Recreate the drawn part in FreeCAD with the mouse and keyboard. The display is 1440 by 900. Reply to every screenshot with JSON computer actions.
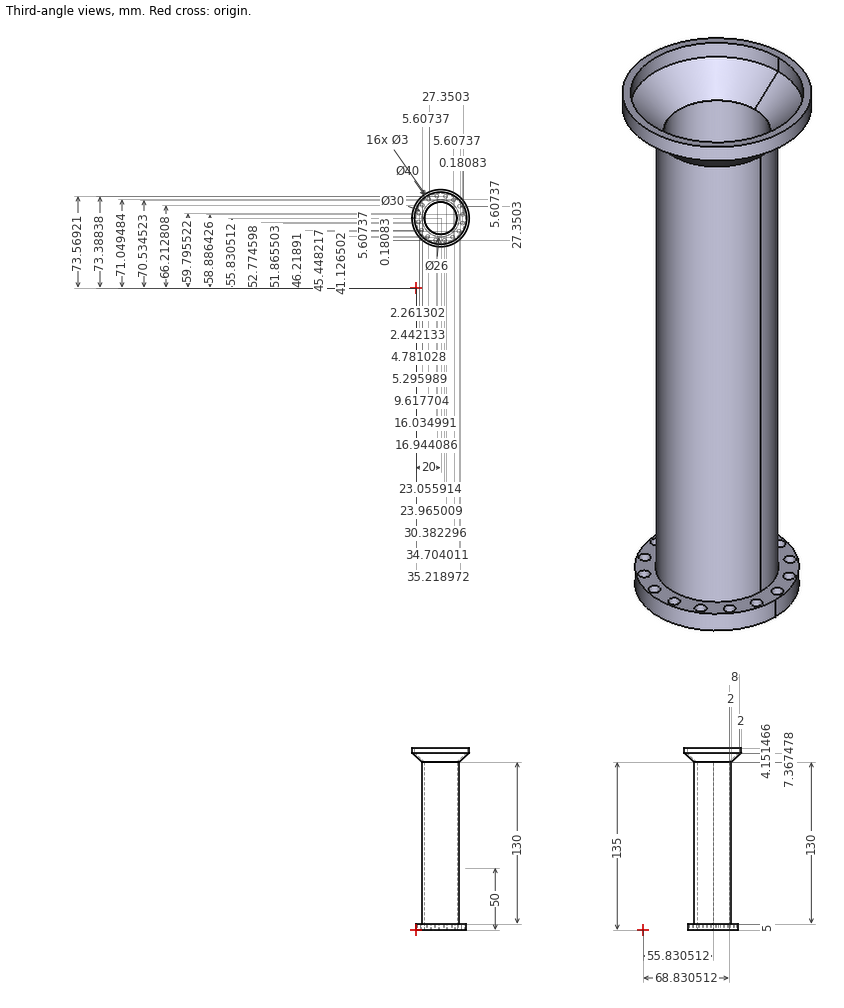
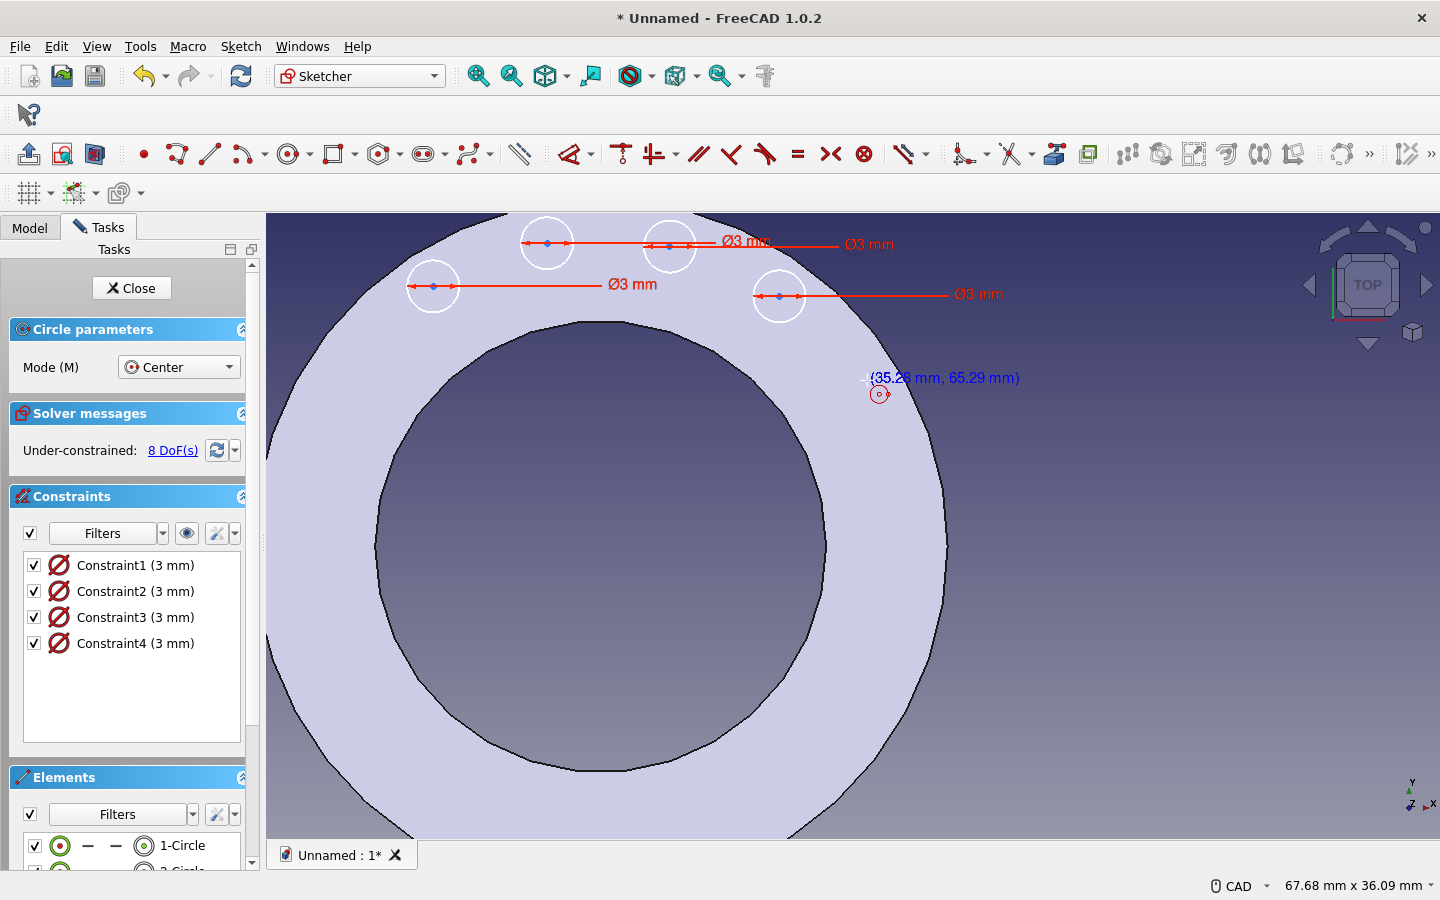
{"action": "scroll", "coordinate": [867, 380], "scroll_direction": "down", "scroll_amount": 6}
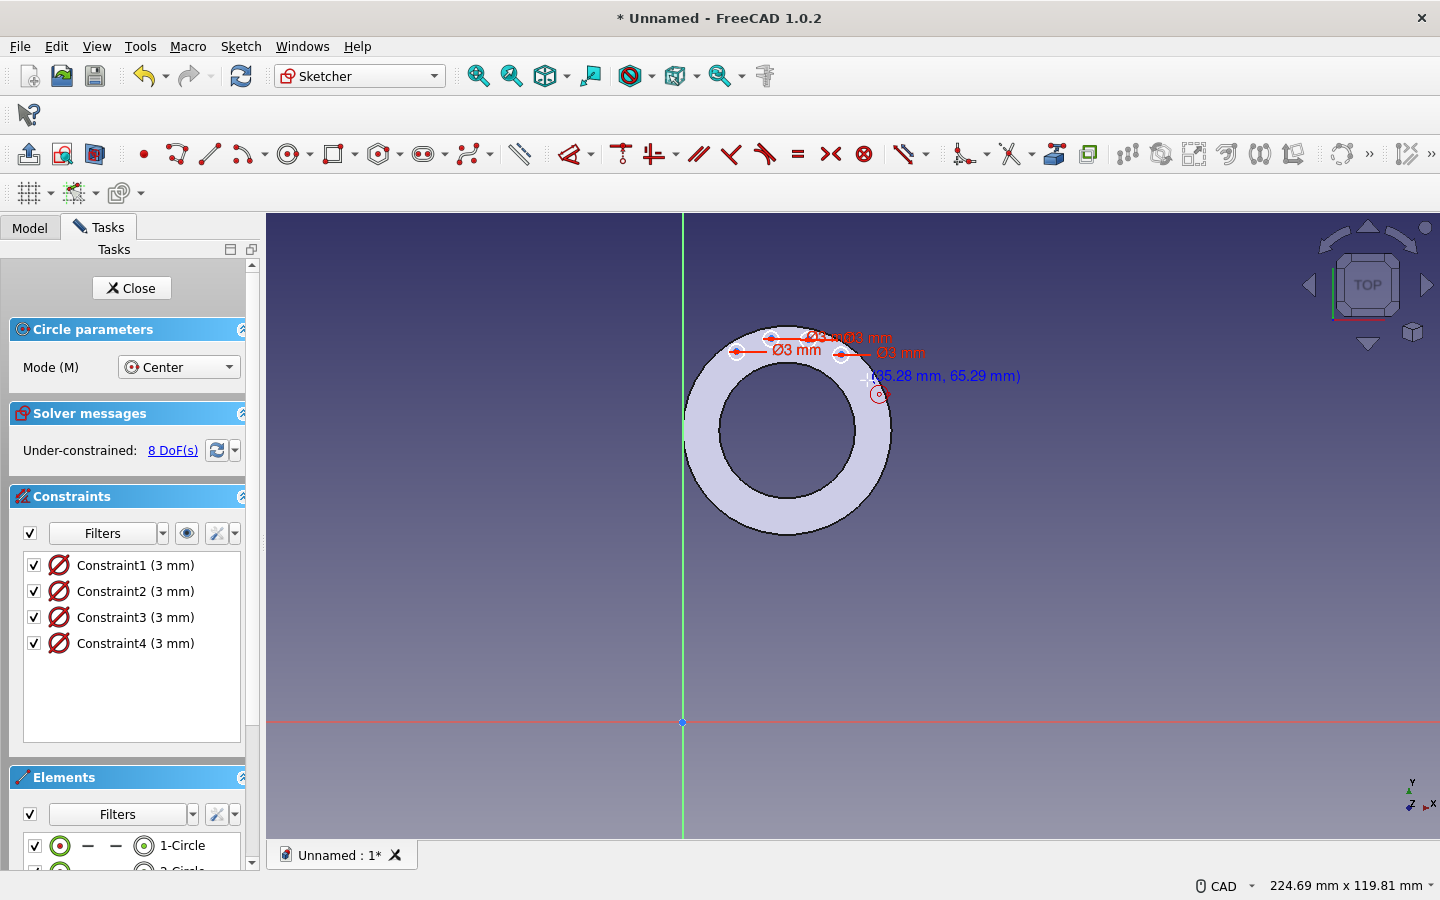
{"action": "left_click", "coordinate": [867, 380]}
{"action": "mouse_move", "coordinate": [872, 375]}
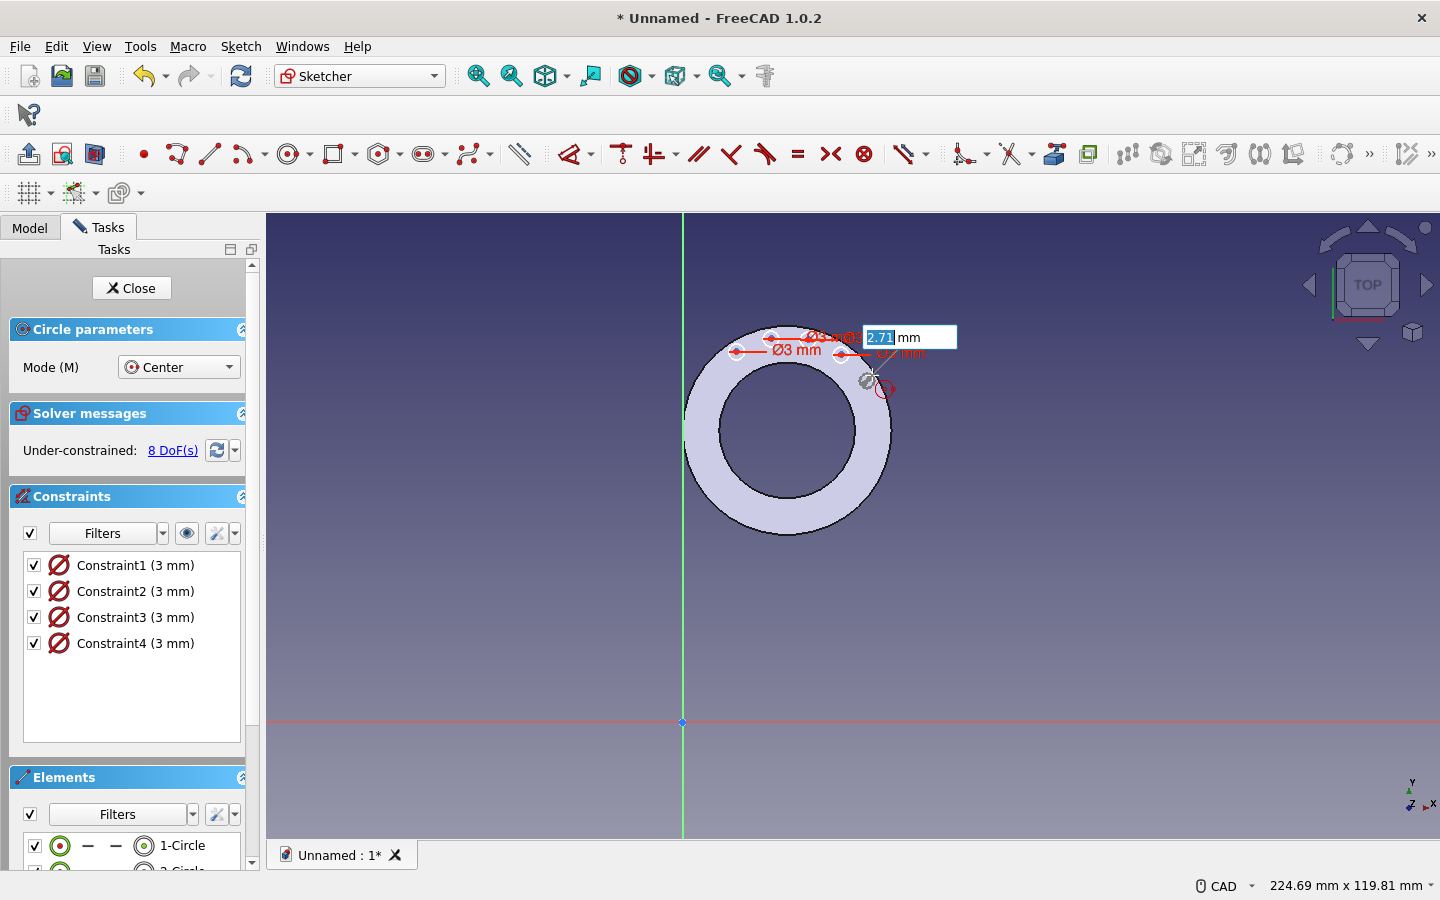
{"action": "type", "text": "3"}
{"action": "key", "text": "Return"}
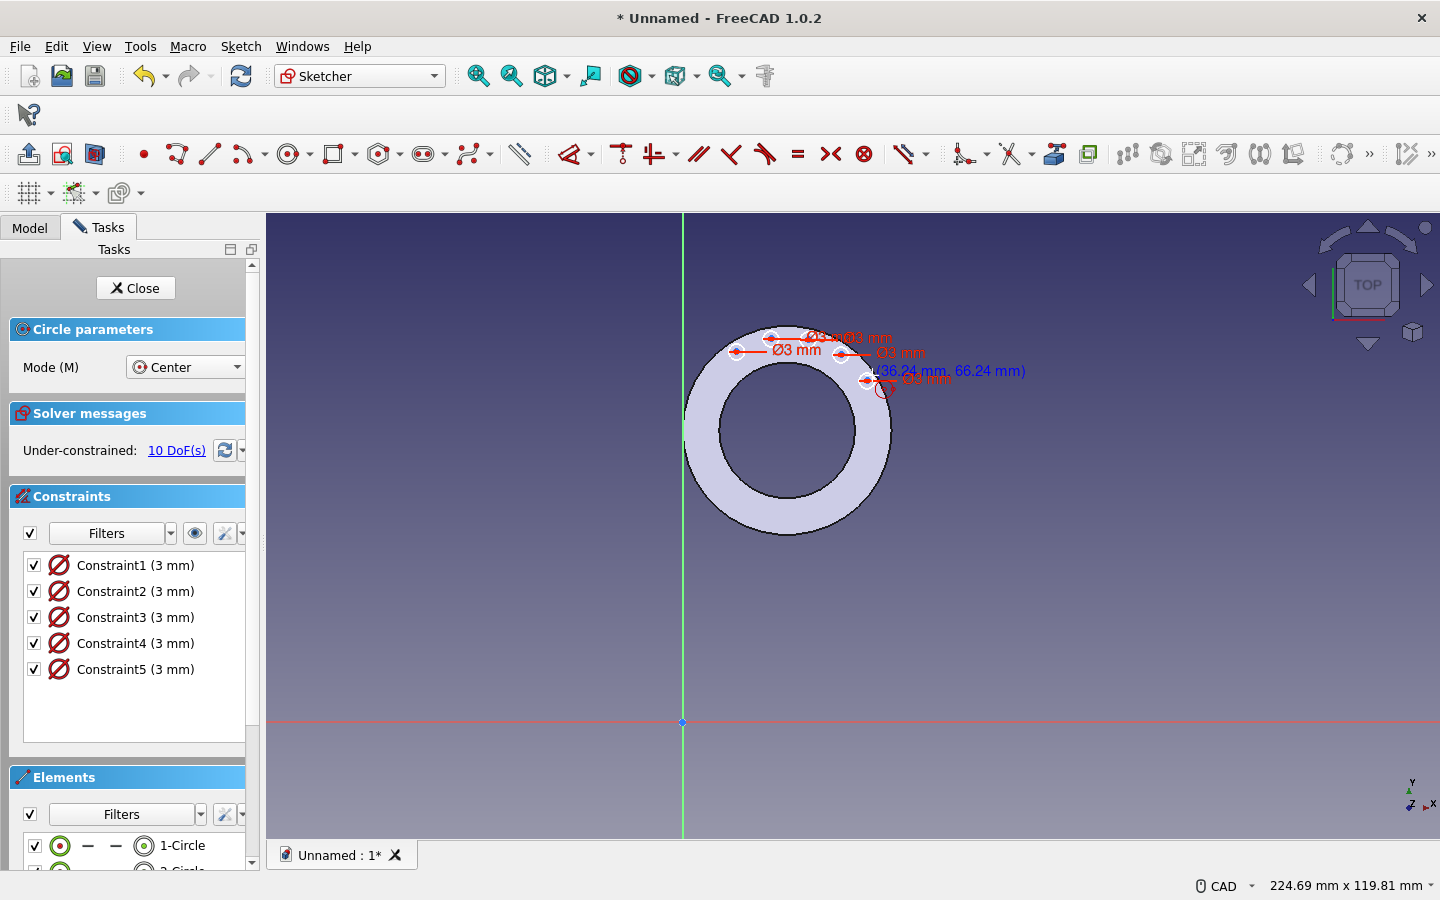
{"action": "scroll", "coordinate": [880, 414], "scroll_direction": "up", "scroll_amount": 6}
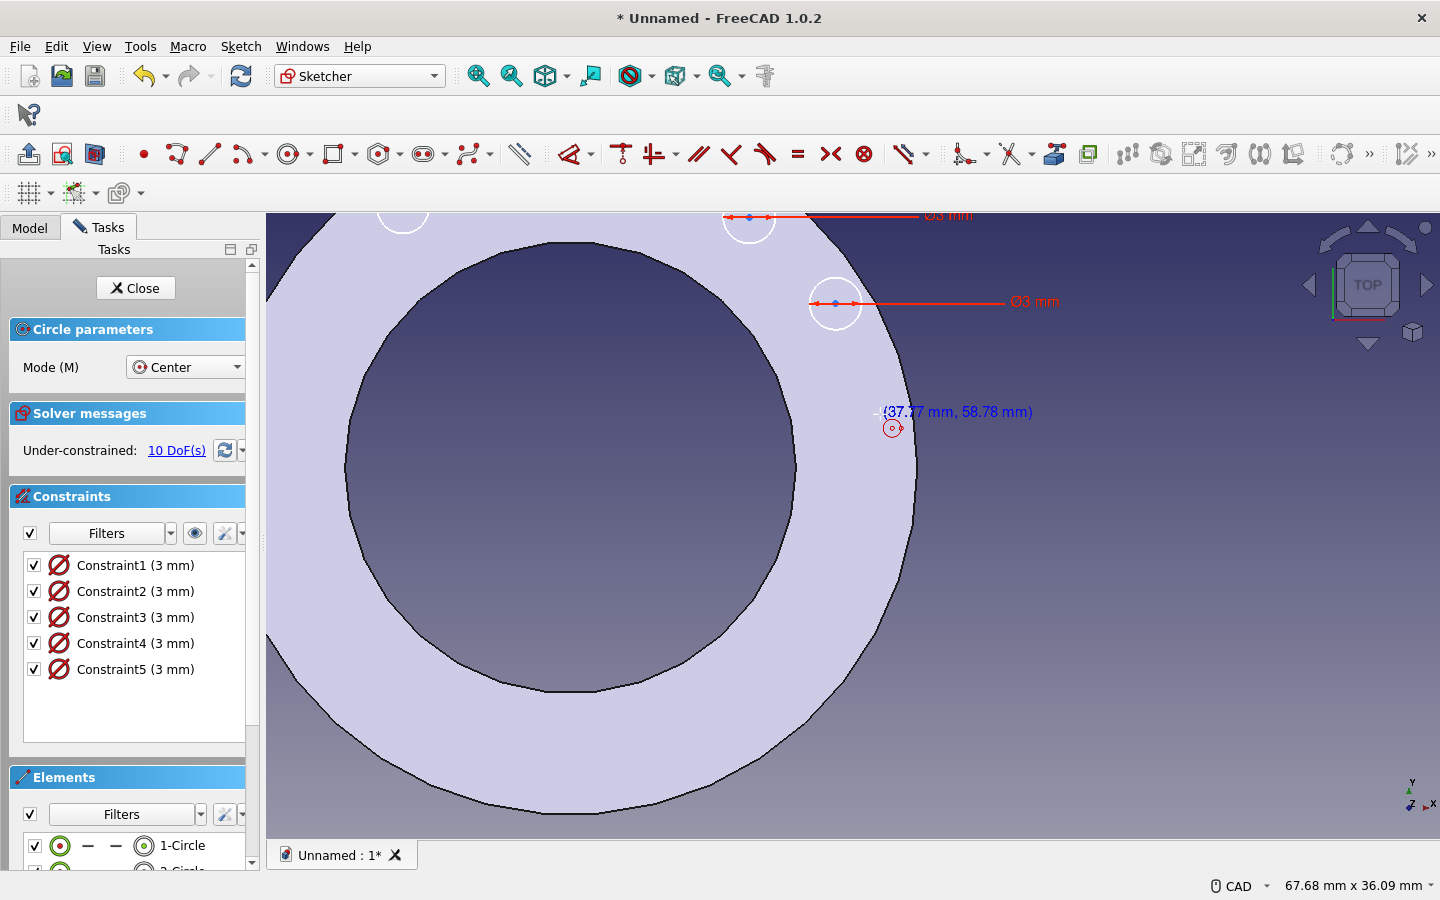
{"action": "scroll", "coordinate": [880, 414], "scroll_direction": "down", "scroll_amount": 6}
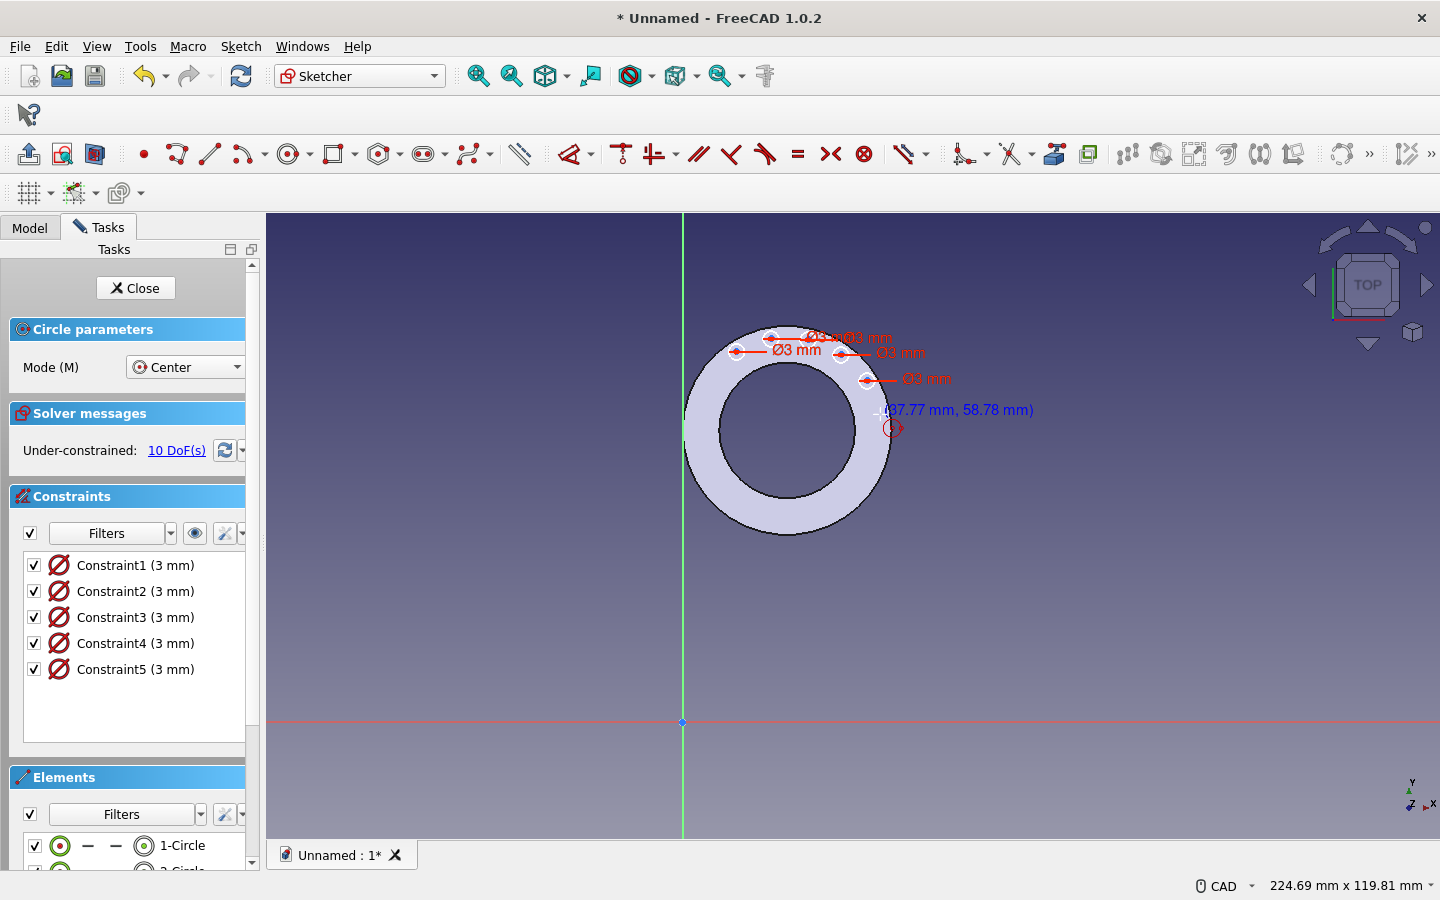
{"action": "left_click", "coordinate": [880, 414]}
{"action": "mouse_move", "coordinate": [885, 409]}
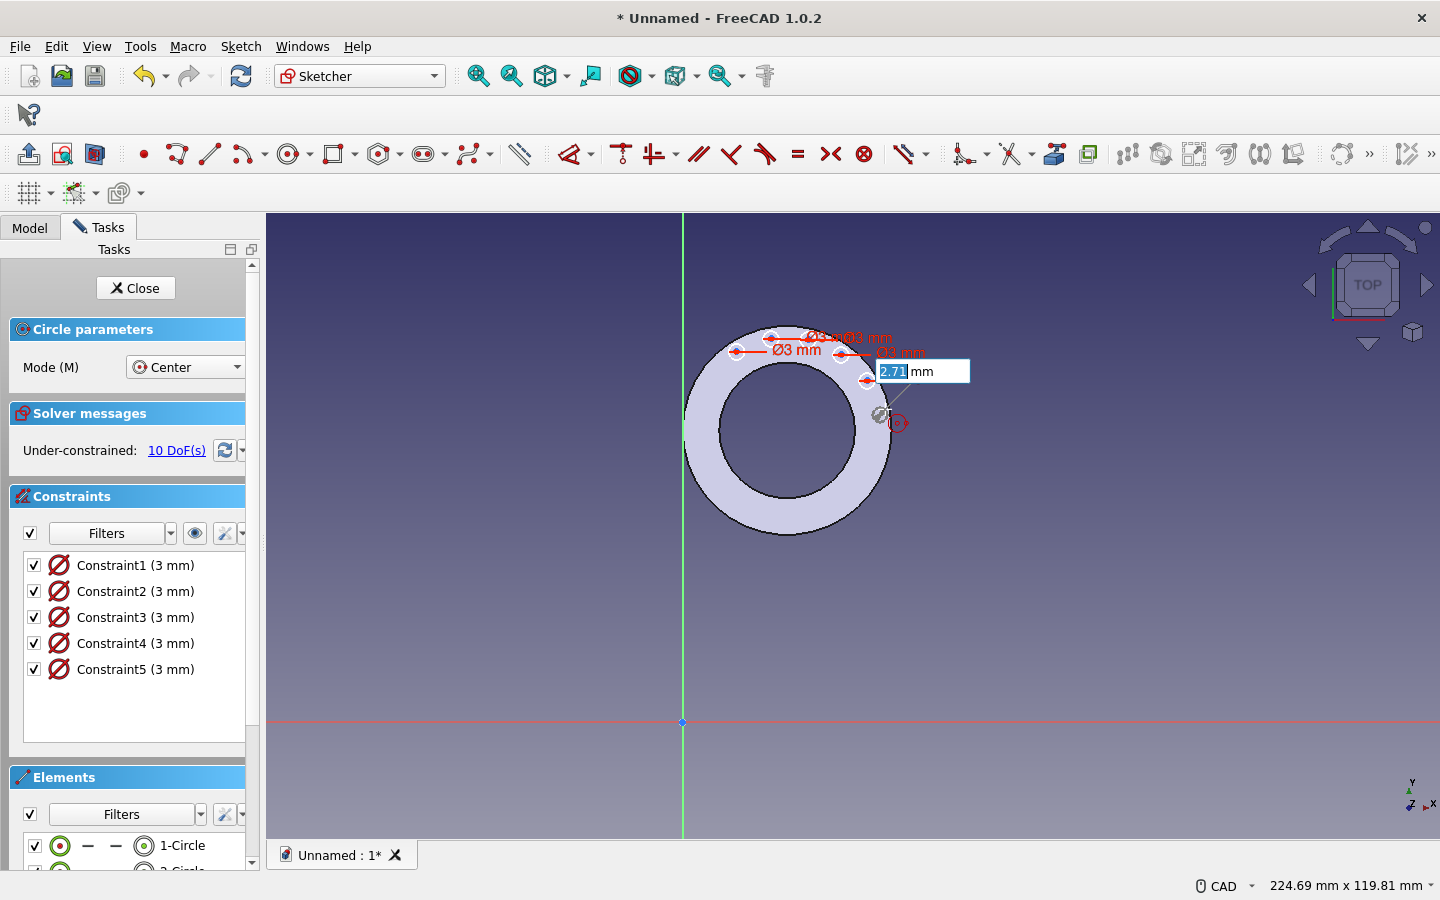
{"action": "type", "text": "3"}
{"action": "key", "text": "Return"}